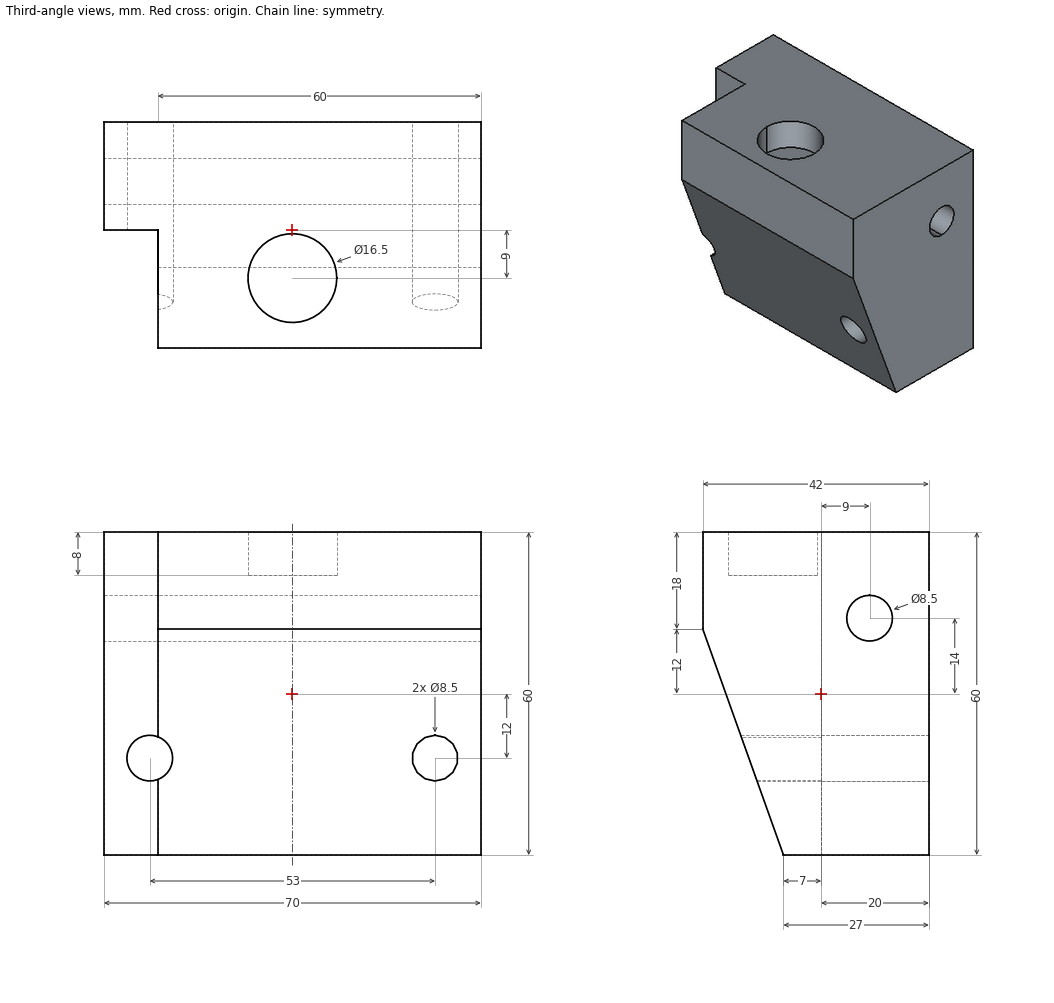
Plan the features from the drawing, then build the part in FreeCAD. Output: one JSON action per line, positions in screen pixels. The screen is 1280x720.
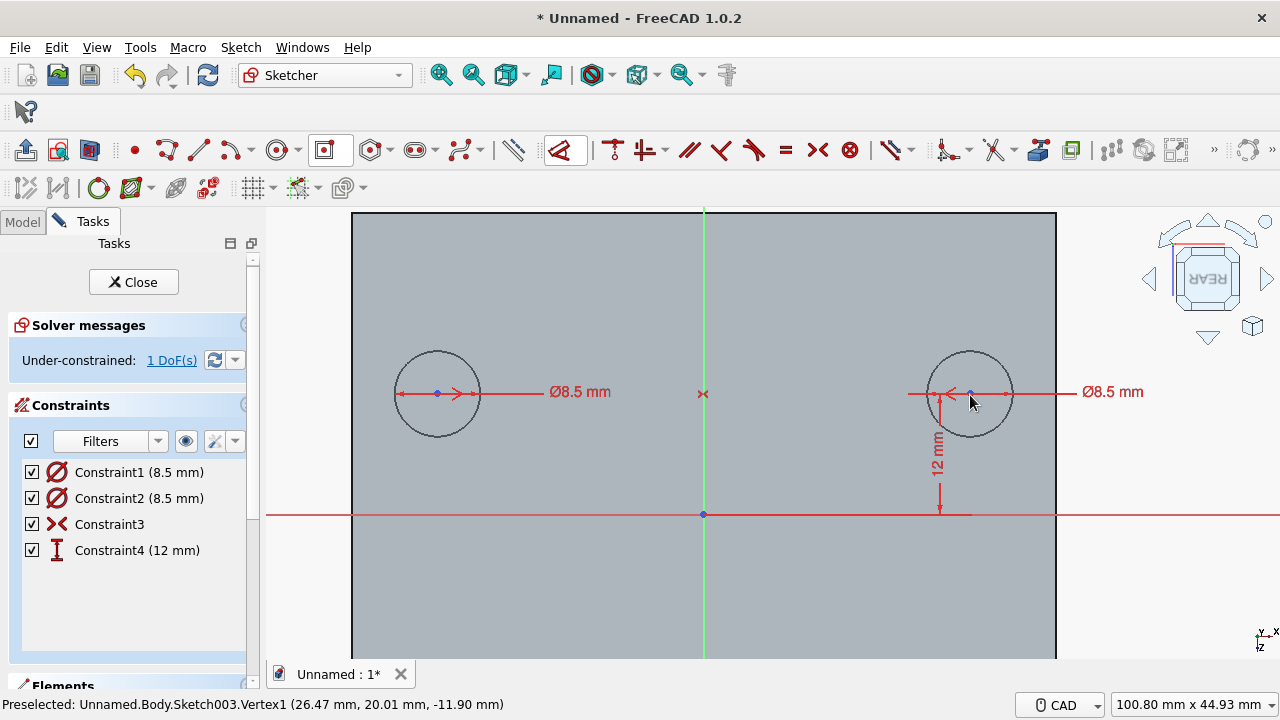
{"action": "left_click", "coordinate": [970, 394]}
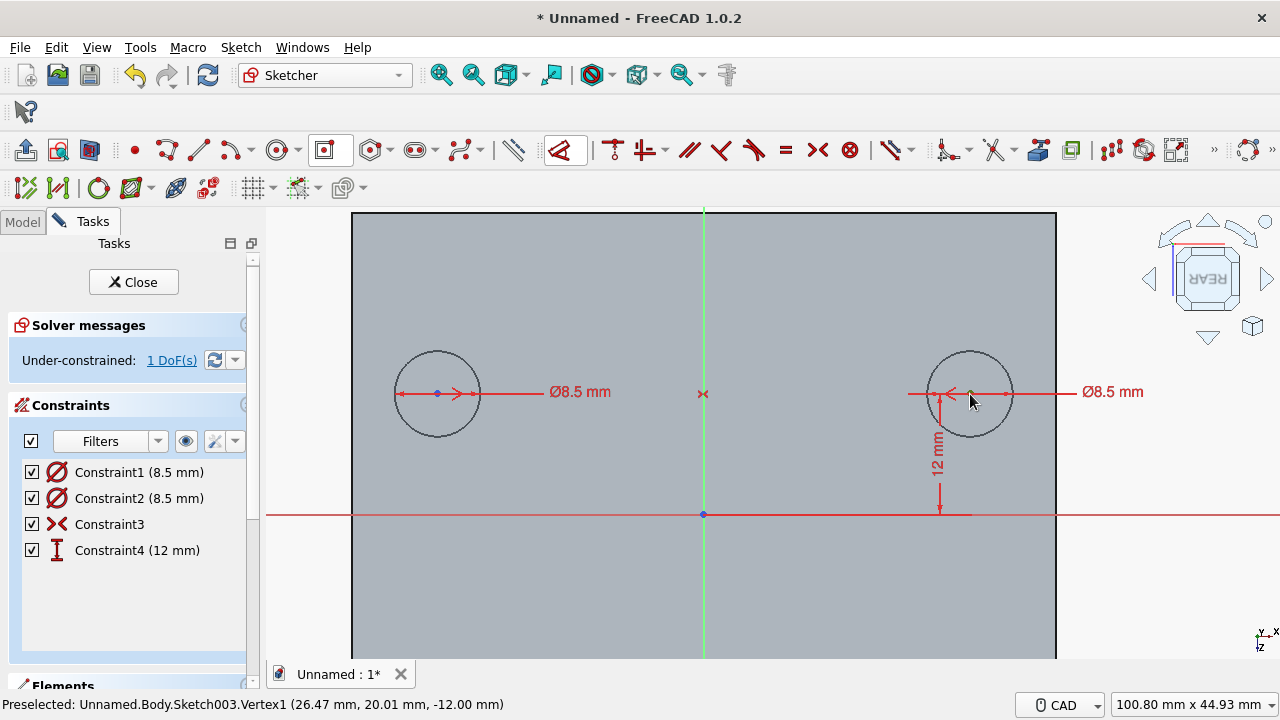
{"action": "left_click", "coordinate": [437, 394]}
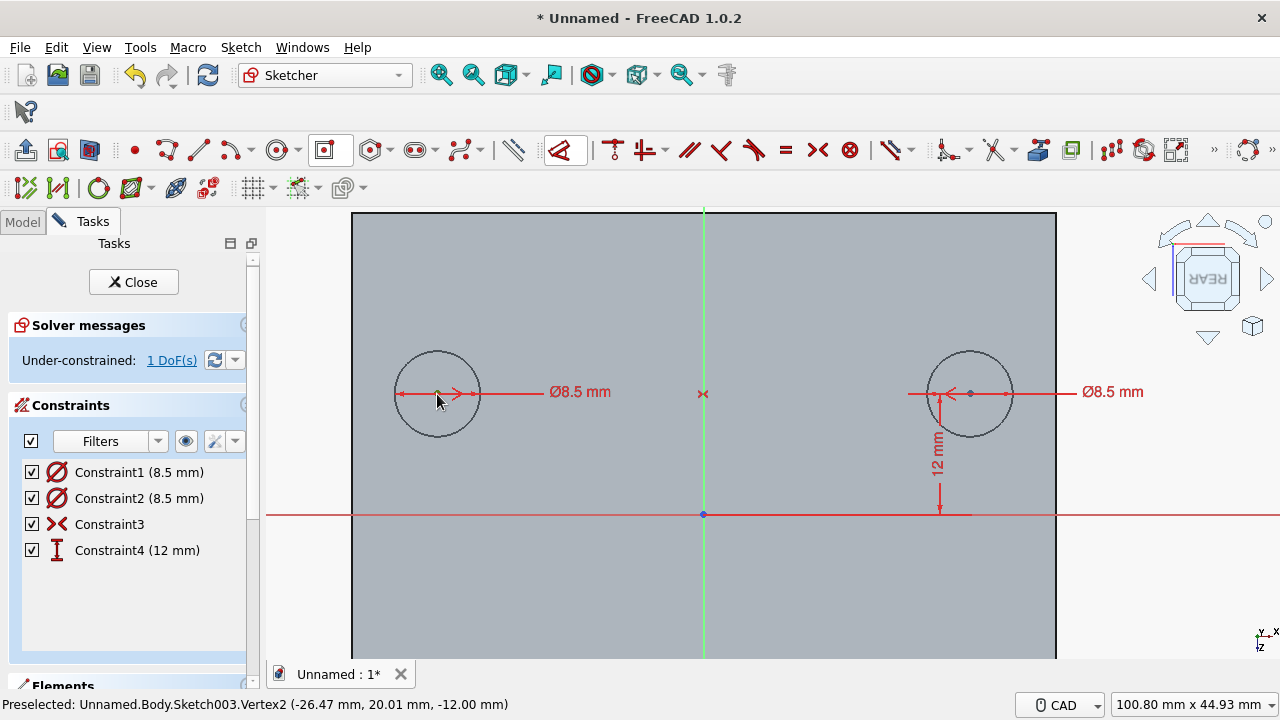
{"action": "key", "text": "l"}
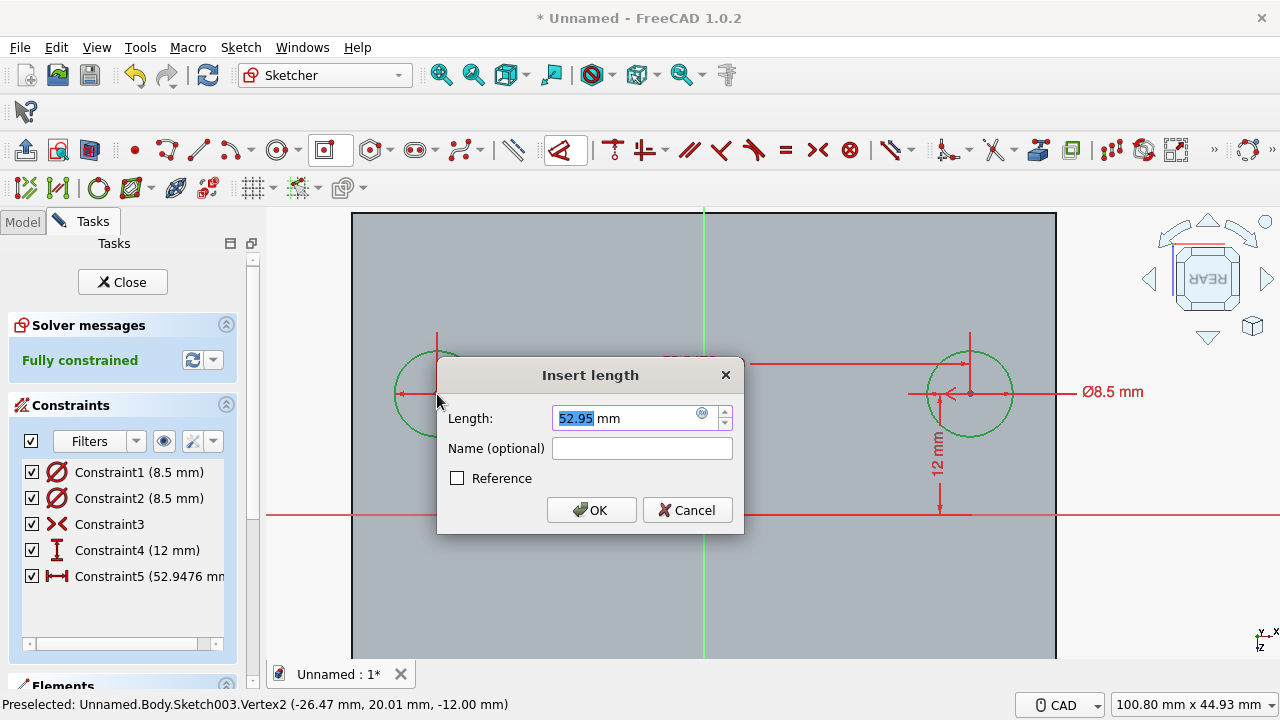
{"action": "type", "text": "53"}
{"action": "key", "text": "Return"}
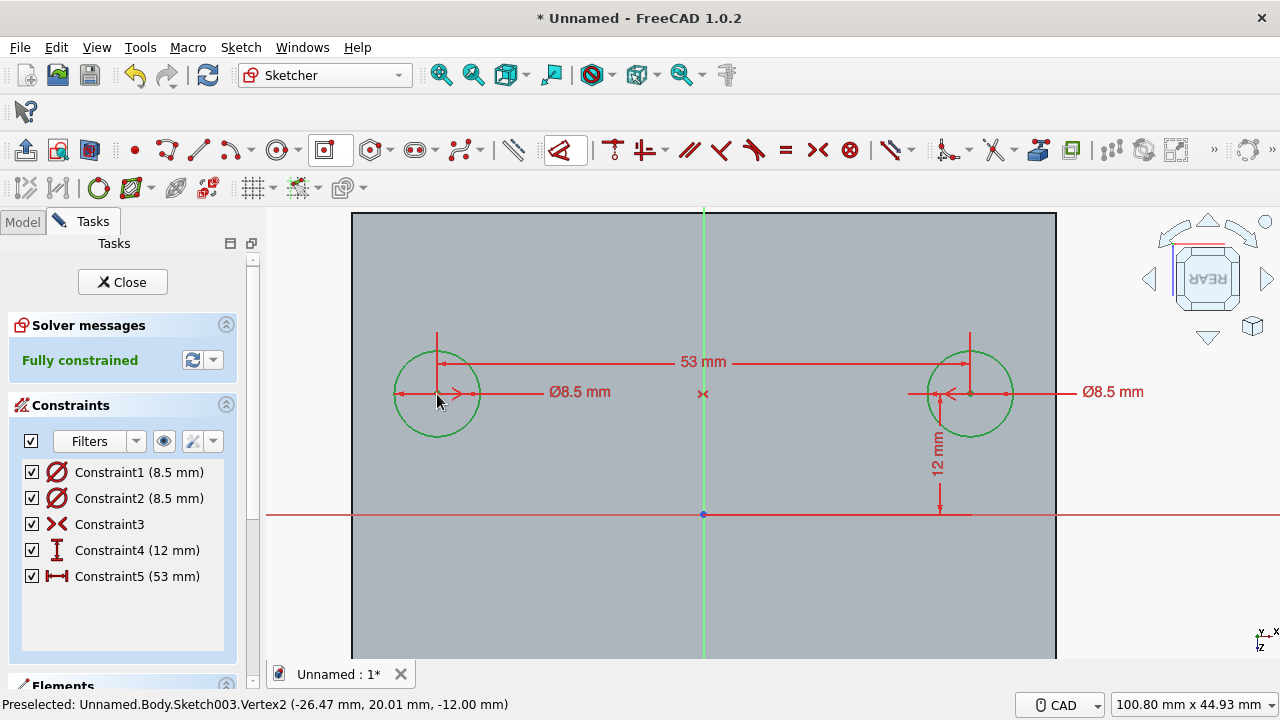
{"action": "left_click", "coordinate": [123, 282]}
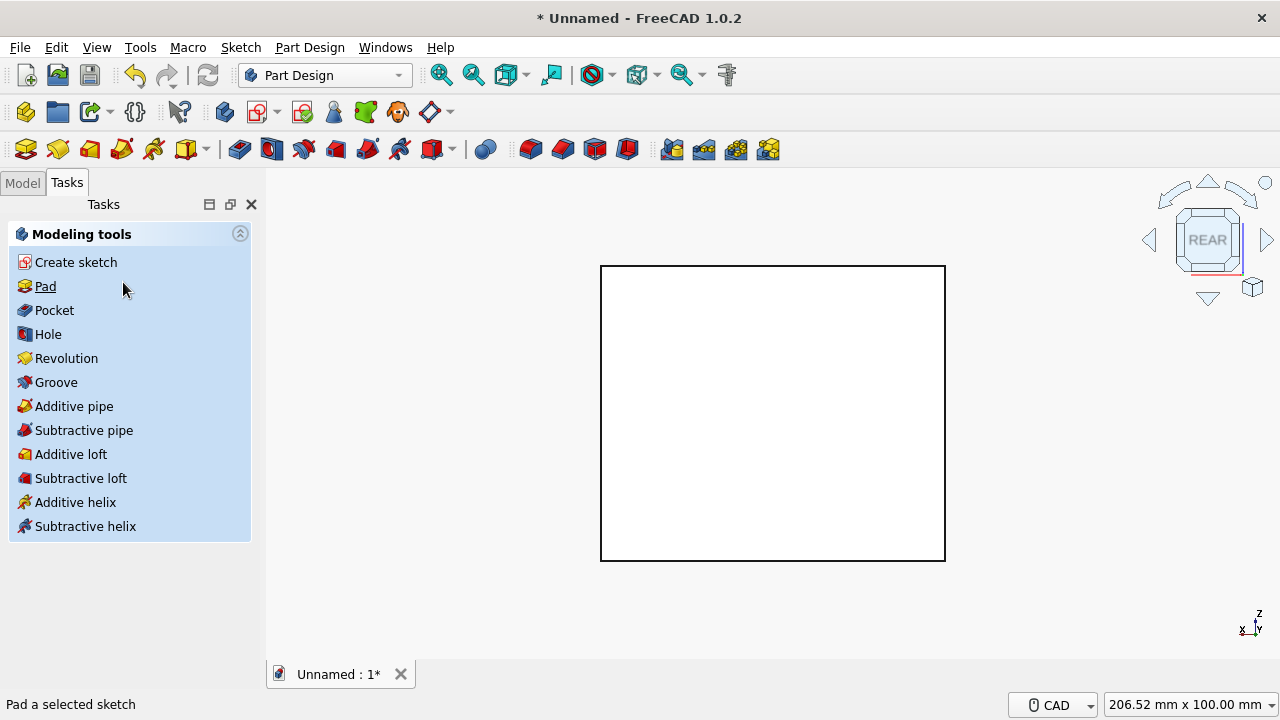
{"action": "left_click", "coordinate": [240, 150]}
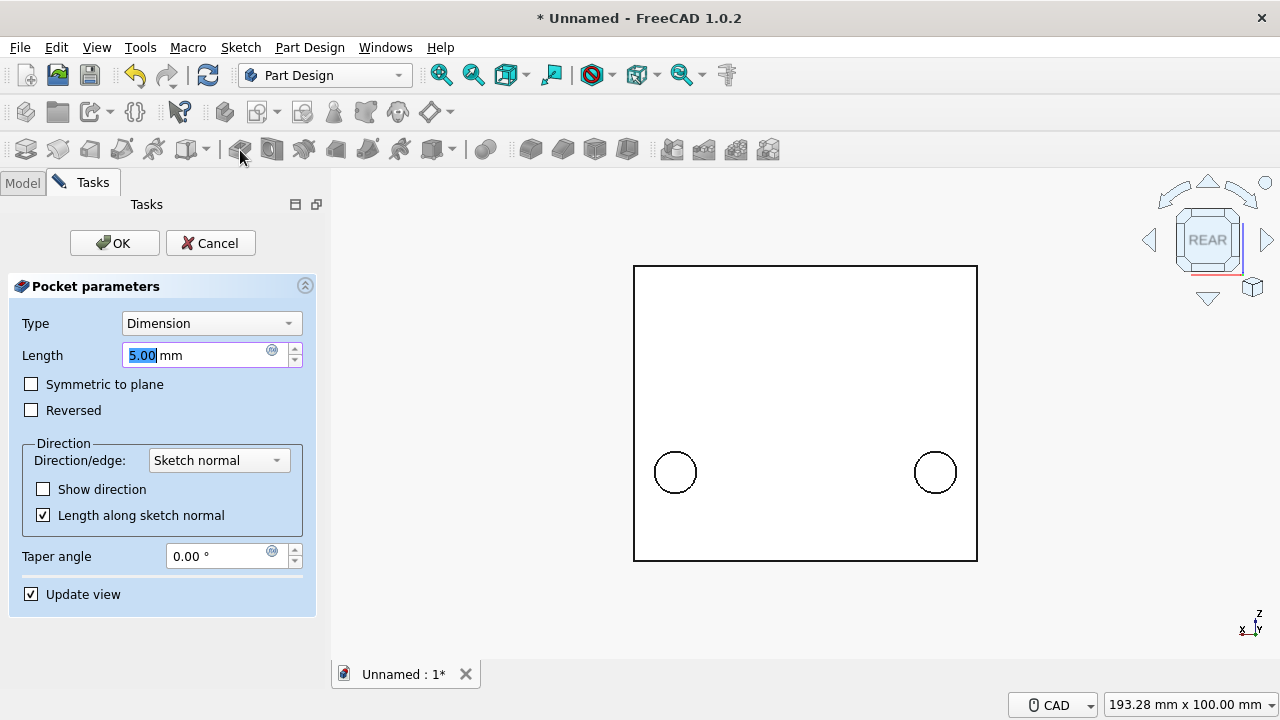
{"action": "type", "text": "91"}
{"action": "key", "text": "Tab"}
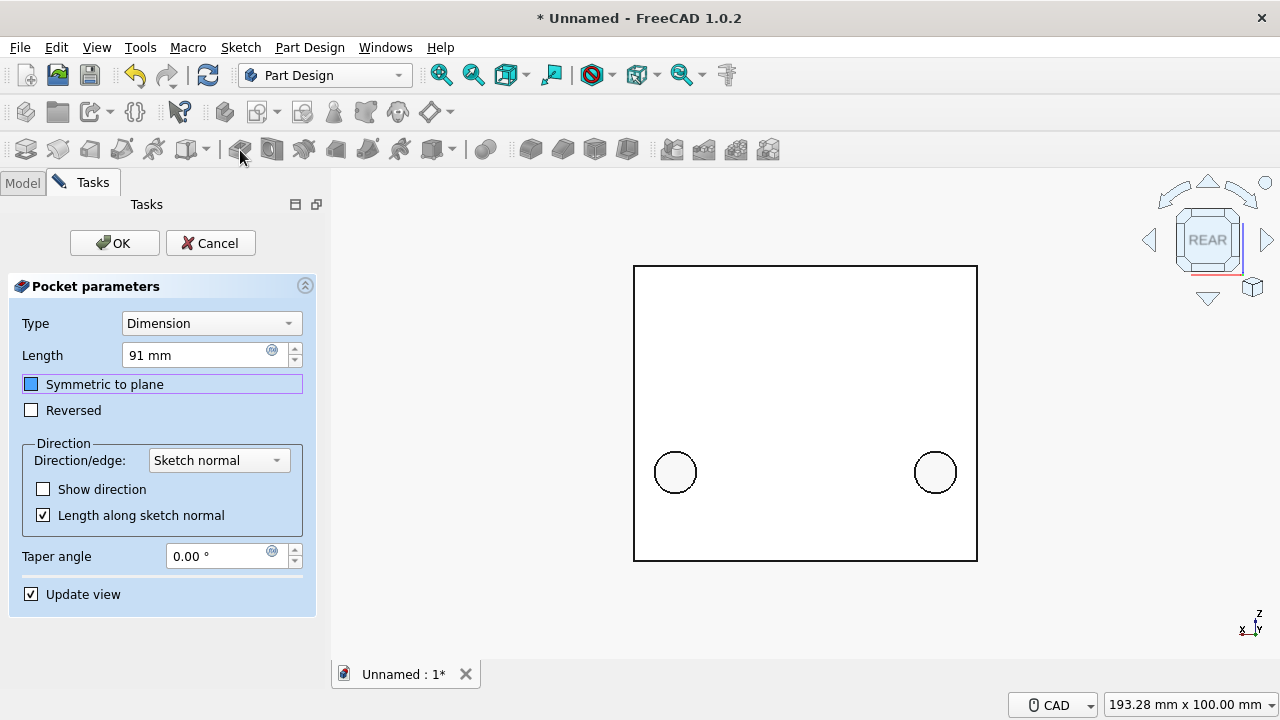
{"action": "left_click", "coordinate": [115, 243]}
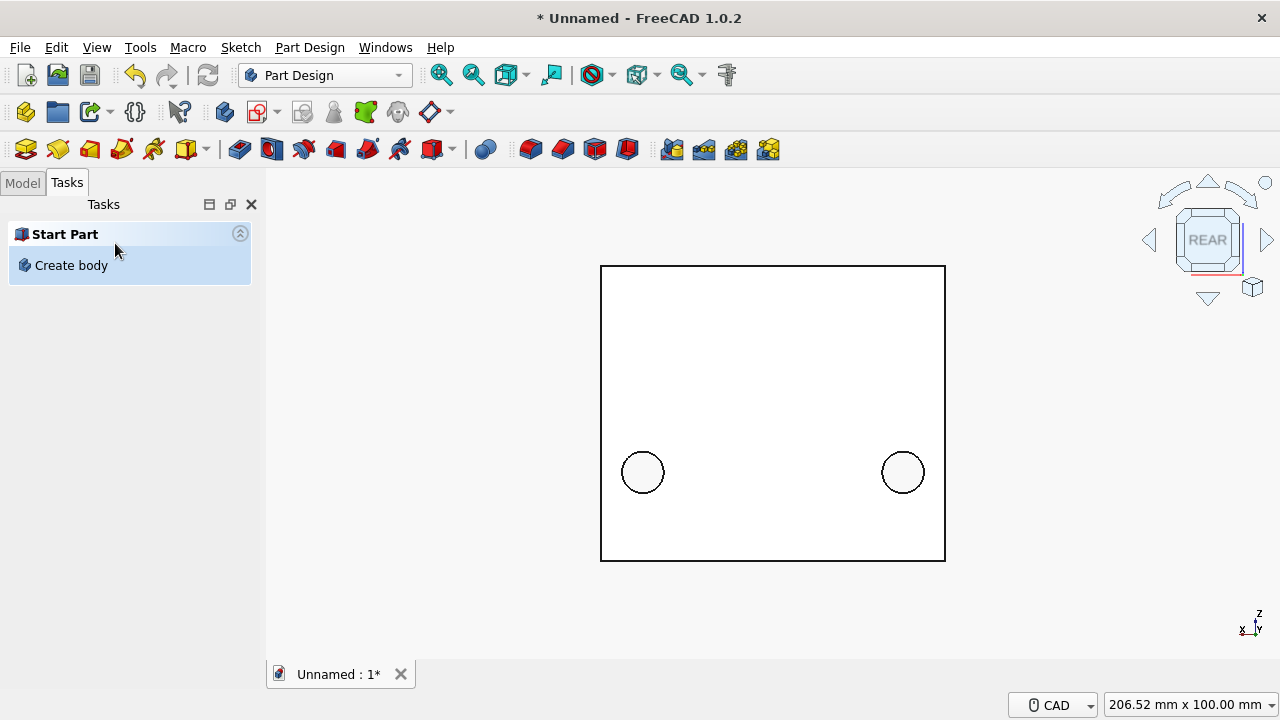
{"action": "key", "text": "0"}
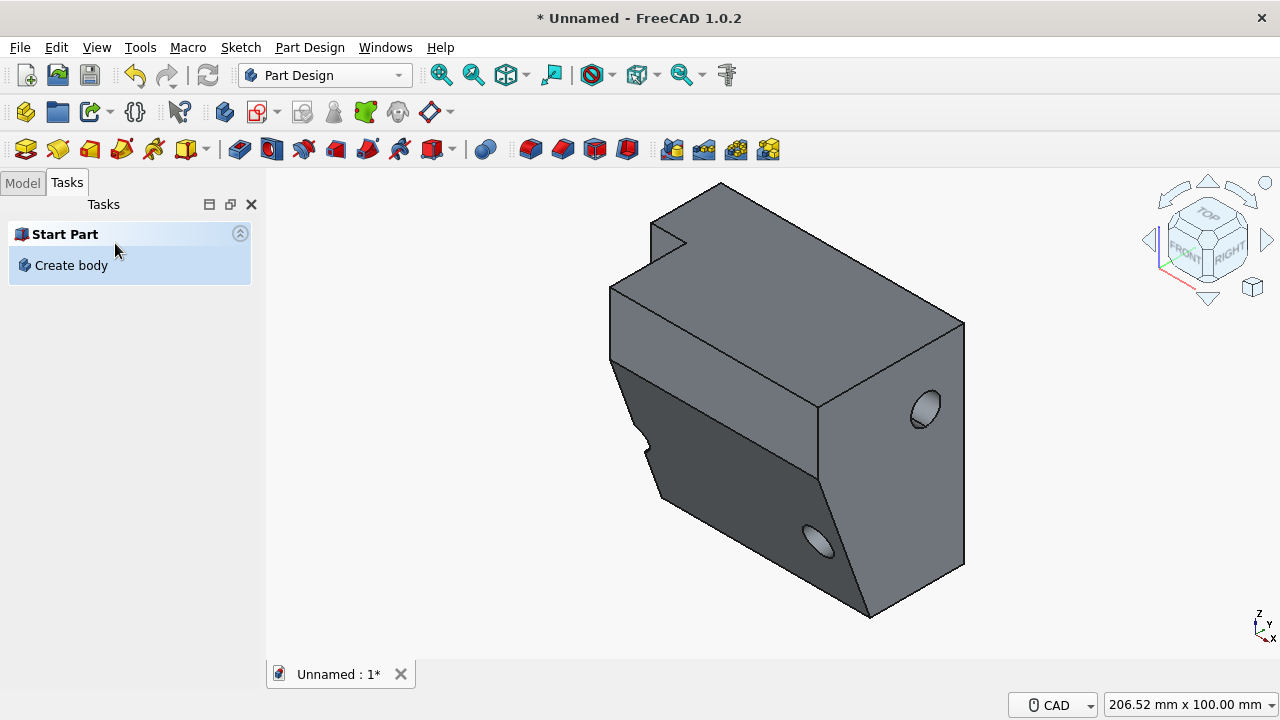
{"action": "left_click", "coordinate": [804, 314]}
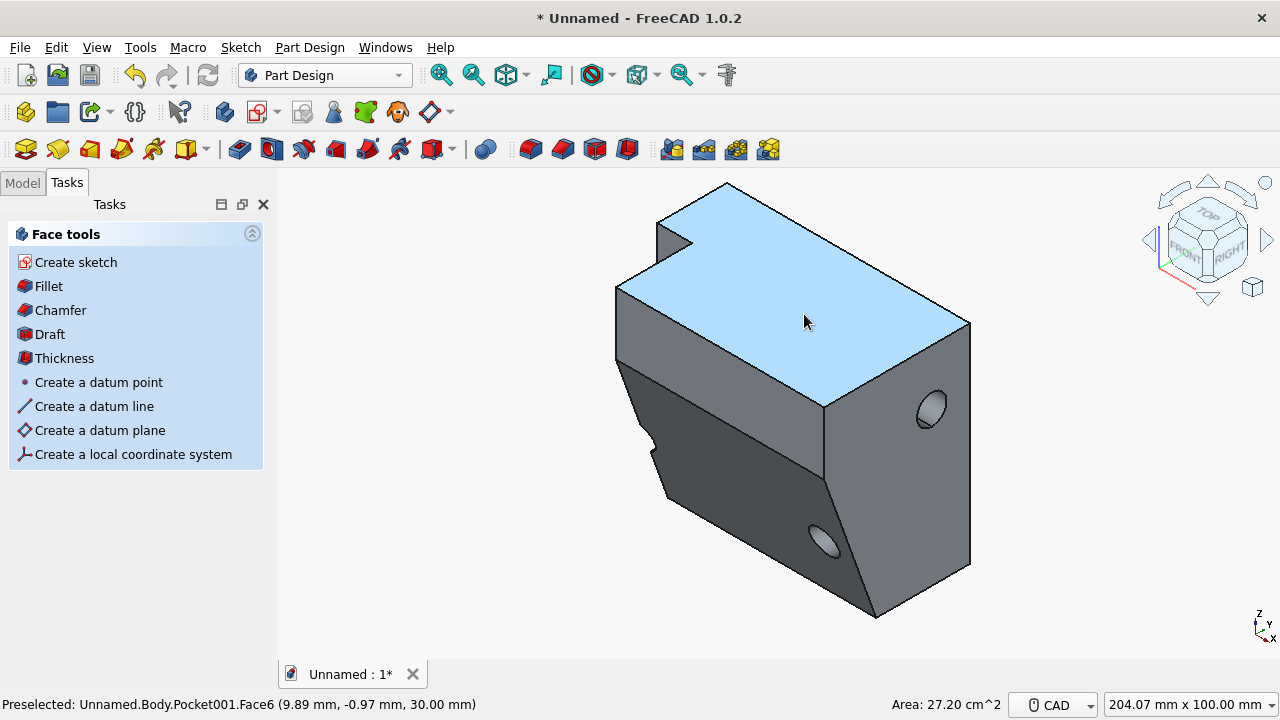
{"action": "left_click", "coordinate": [258, 112]}